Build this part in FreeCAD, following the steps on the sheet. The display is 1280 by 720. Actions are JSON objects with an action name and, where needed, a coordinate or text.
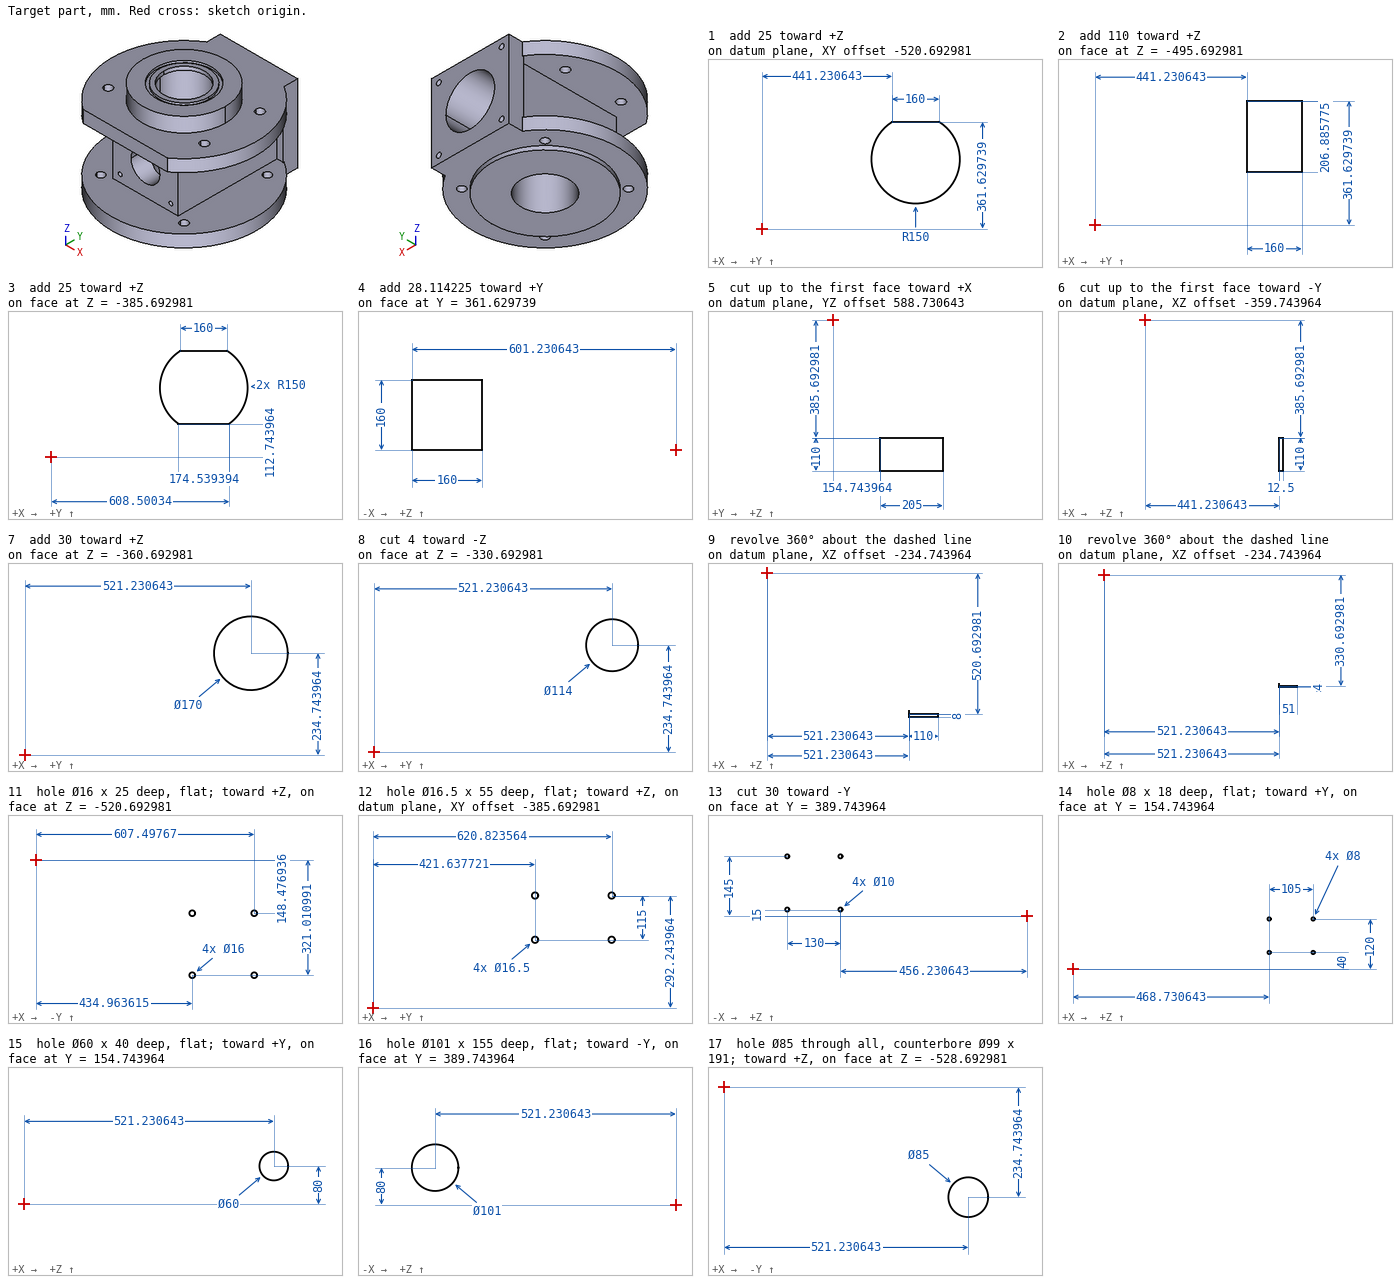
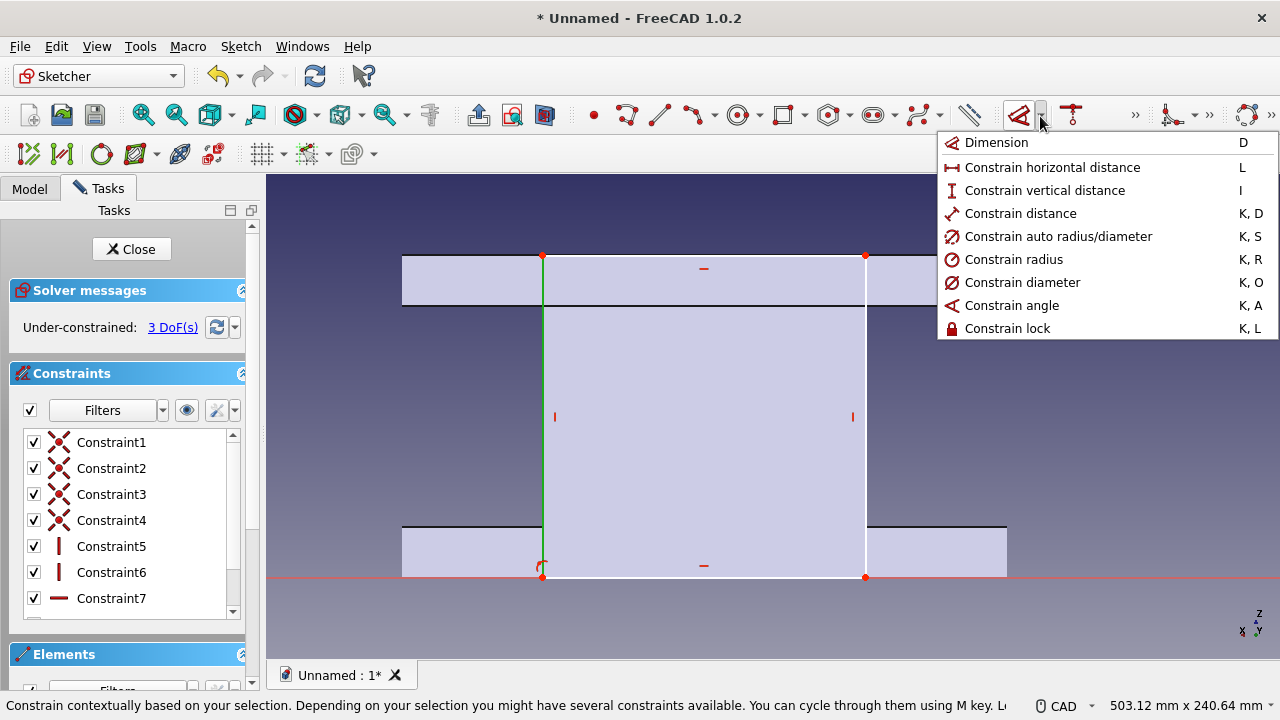
{"action": "left_click", "coordinate": [1108, 190]}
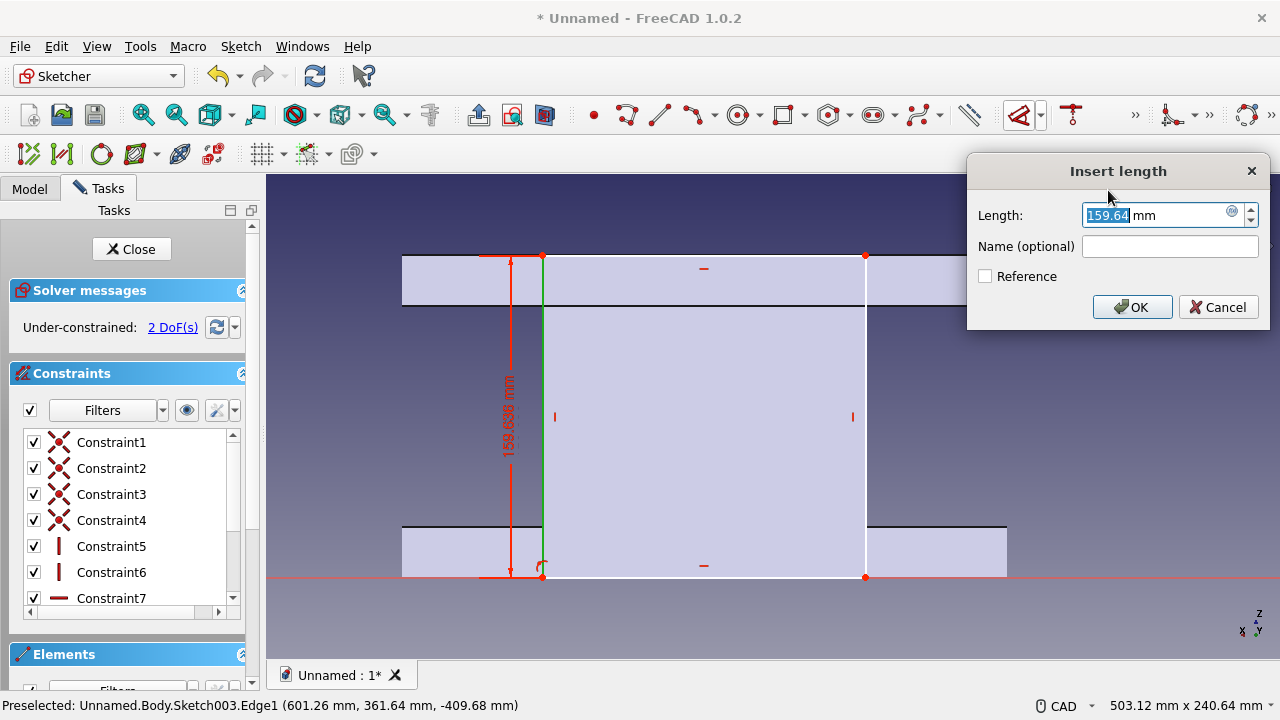
{"action": "type", "text": "160"}
{"action": "key", "text": "Return"}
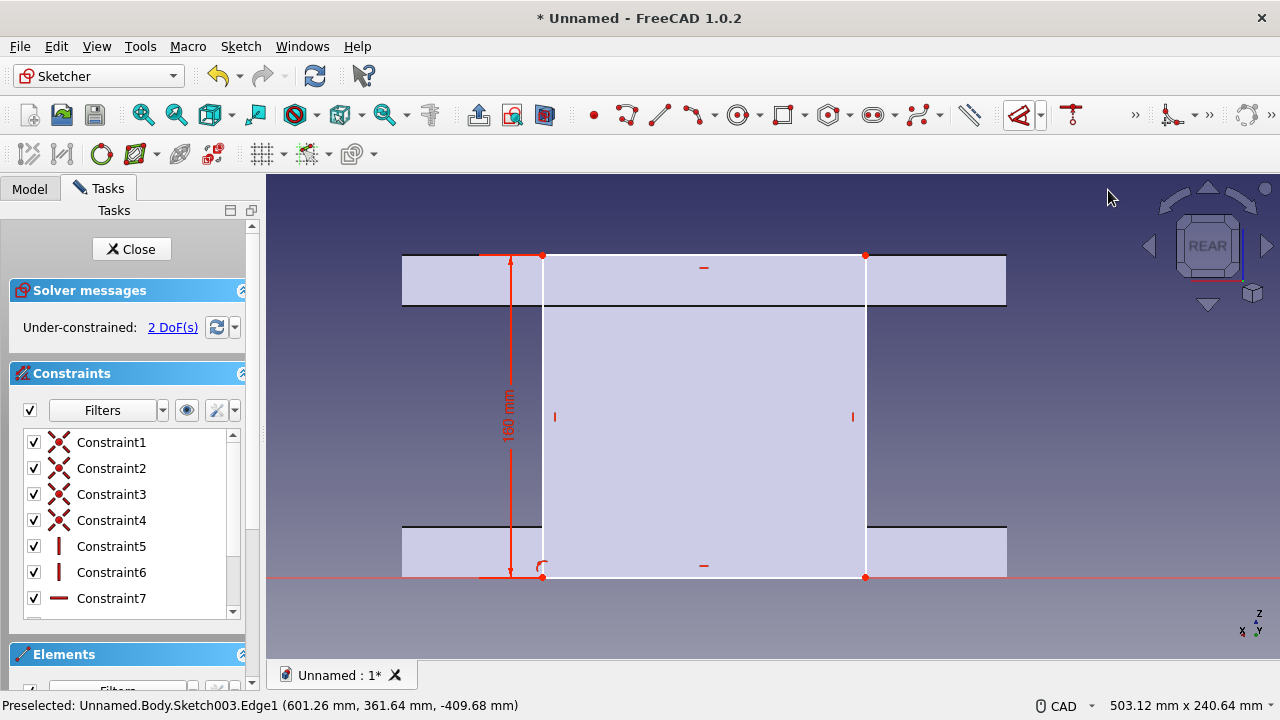
{"action": "left_click", "coordinate": [640, 578]}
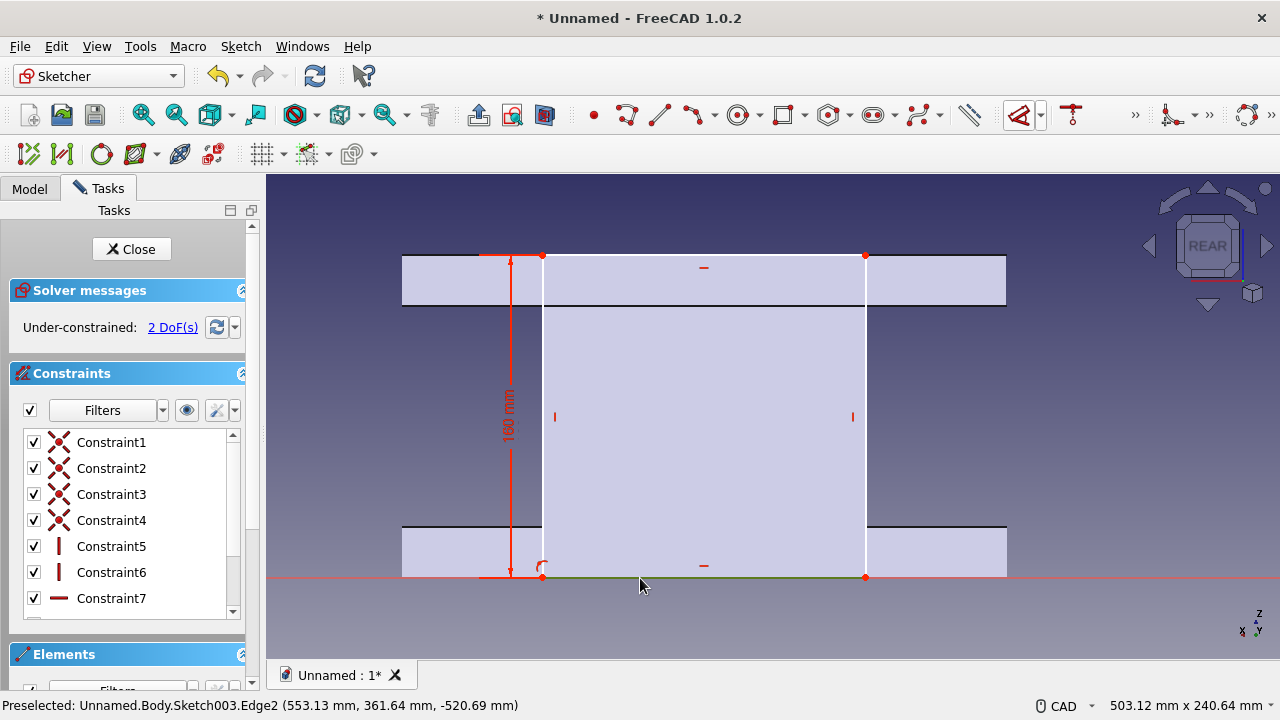
{"action": "left_click", "coordinate": [1040, 116]}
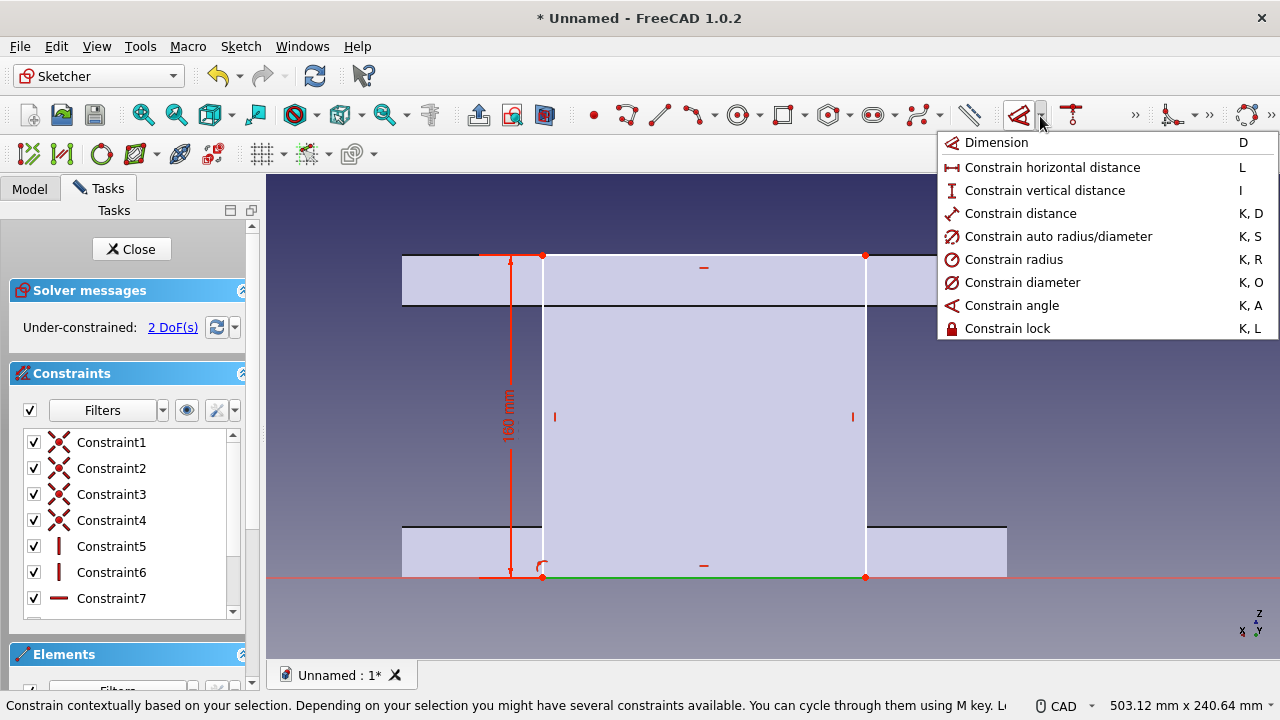
{"action": "left_click", "coordinate": [1108, 168]}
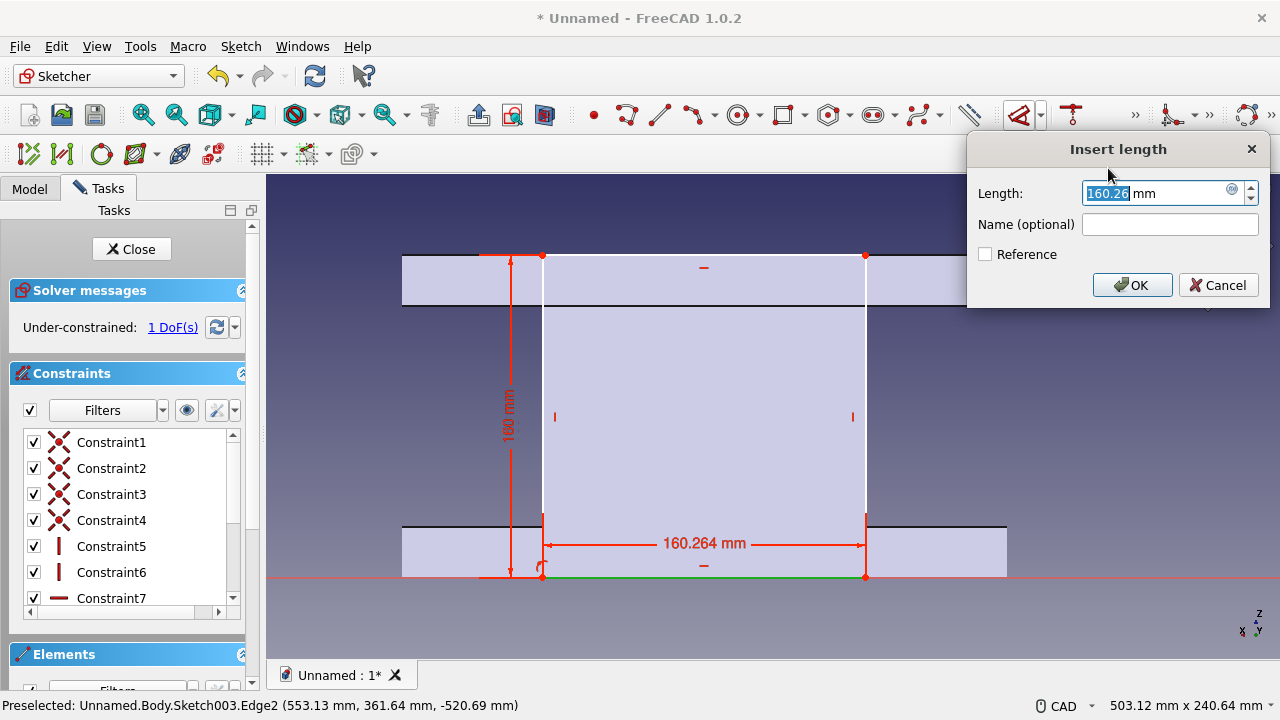
{"action": "type", "text": "160"}
{"action": "key", "text": "Return"}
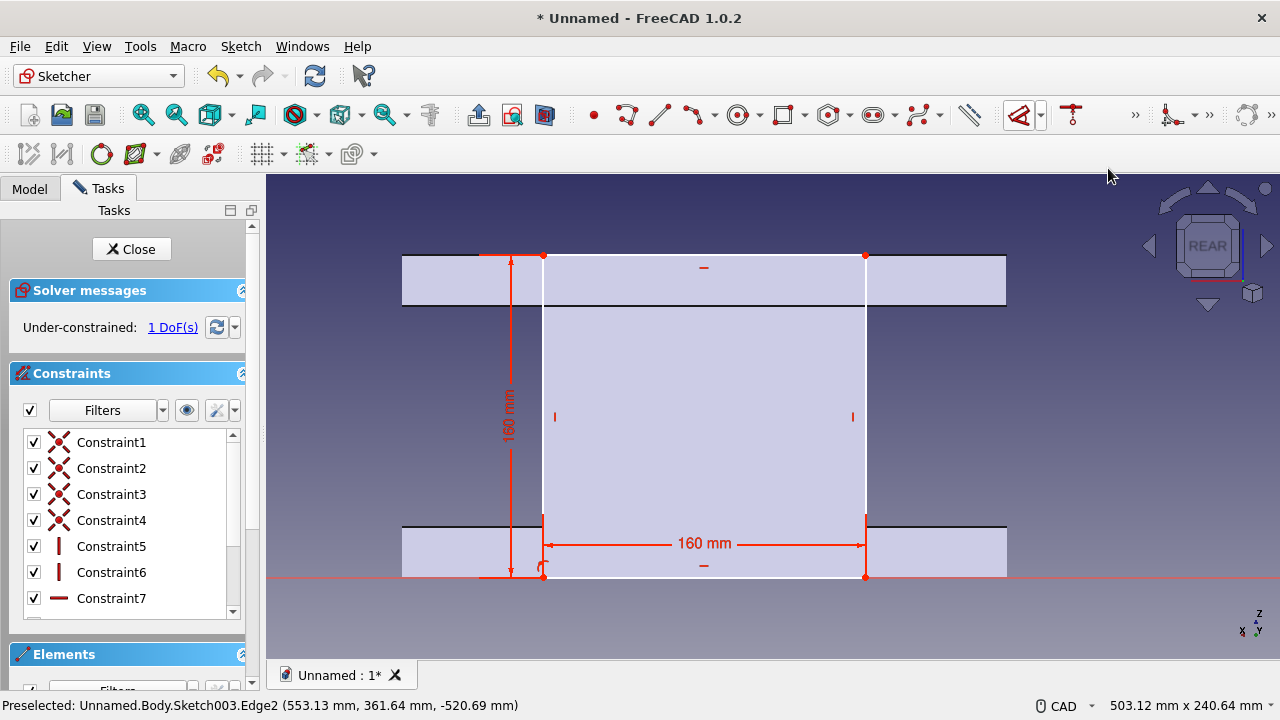
{"action": "left_click", "coordinate": [543, 255]}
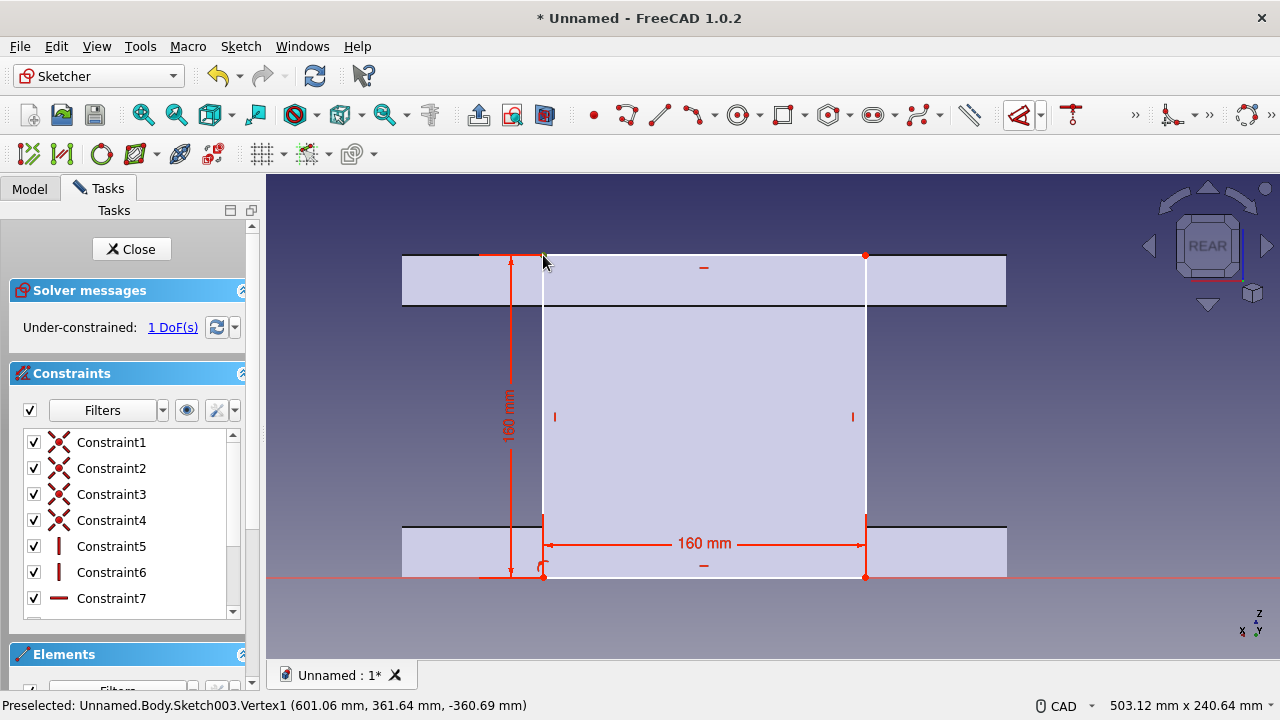
{"action": "key", "text": "l"}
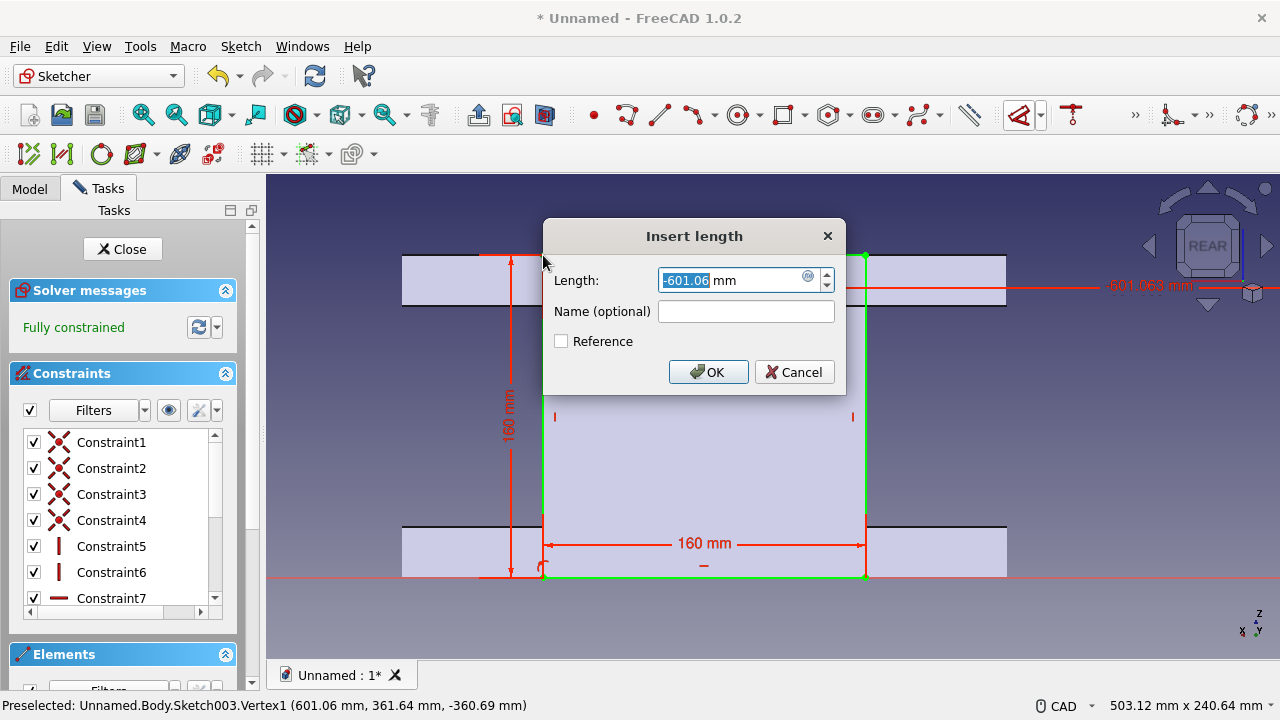
{"action": "type", "text": "-601.230643"}
{"action": "key", "text": "Return"}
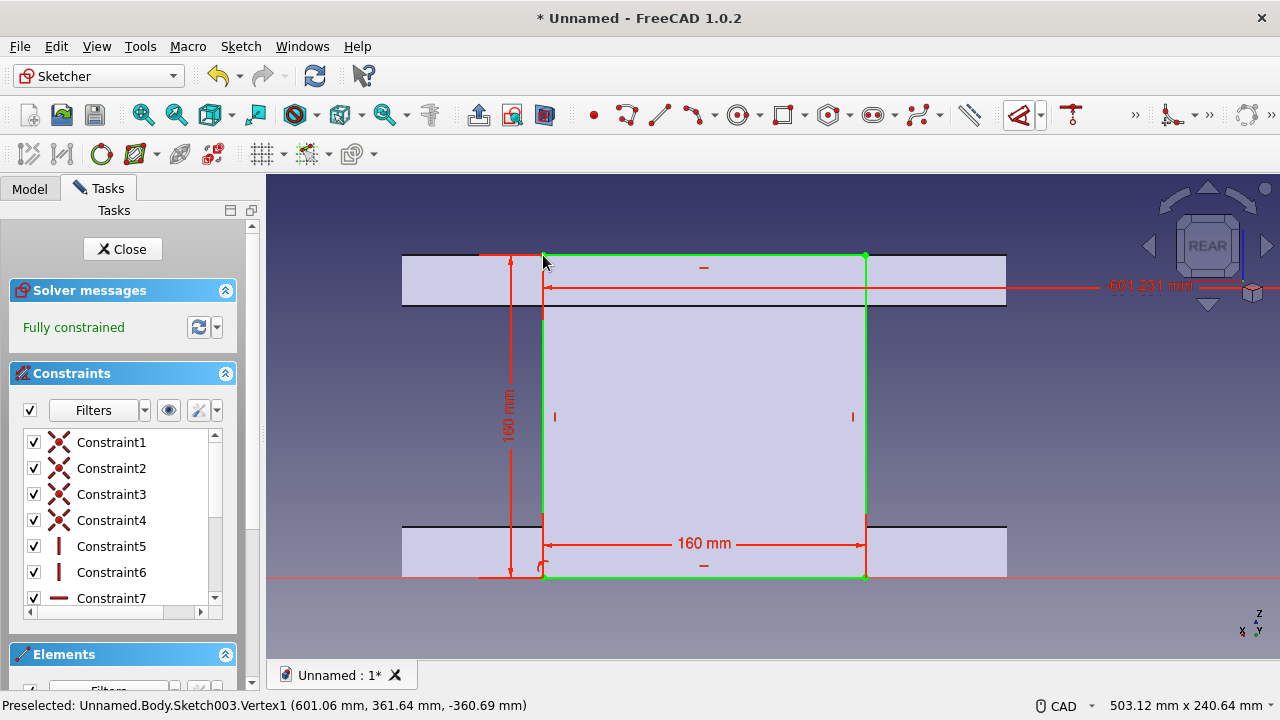
{"action": "left_click", "coordinate": [123, 249]}